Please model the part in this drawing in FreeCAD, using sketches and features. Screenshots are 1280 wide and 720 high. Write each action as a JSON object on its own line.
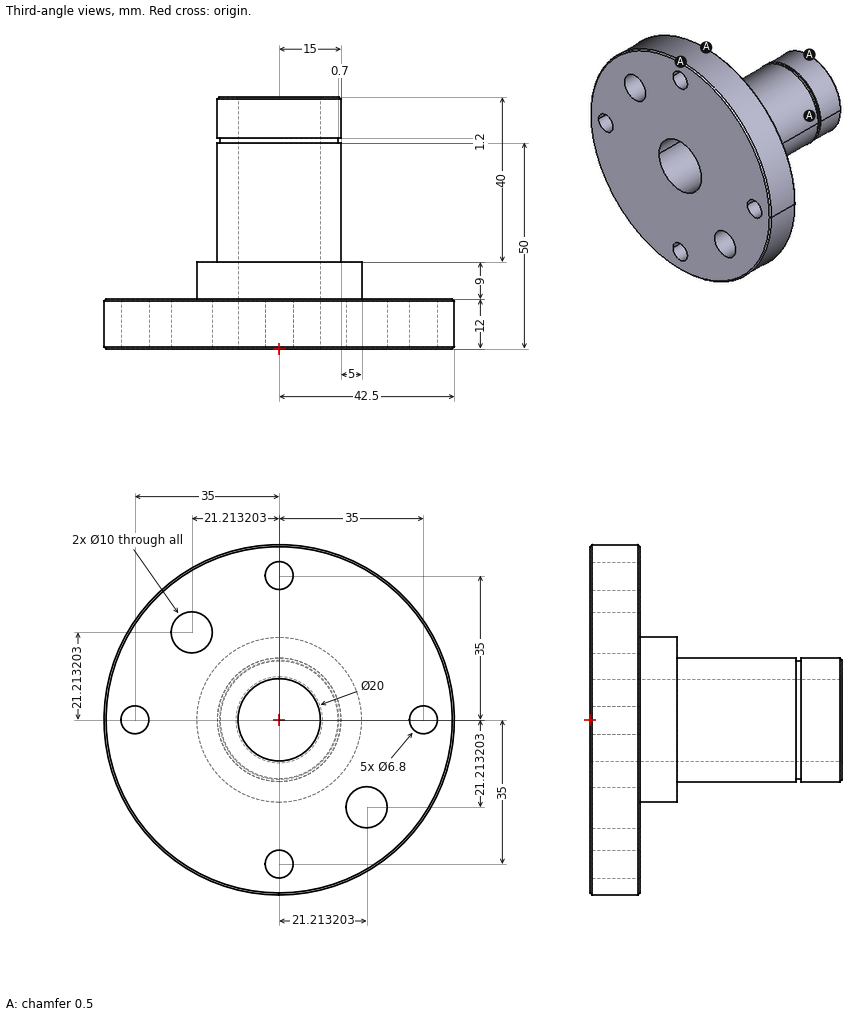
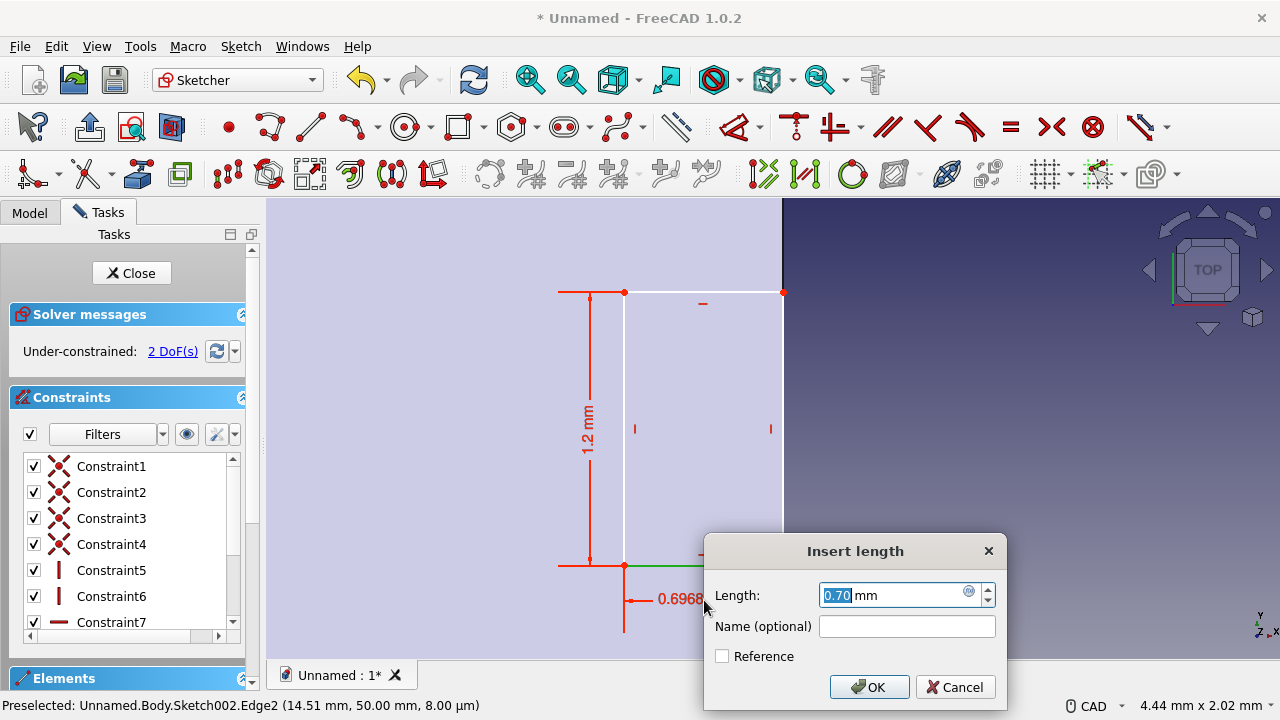
{"action": "type", "text": "0.7"}
{"action": "key", "text": "Return"}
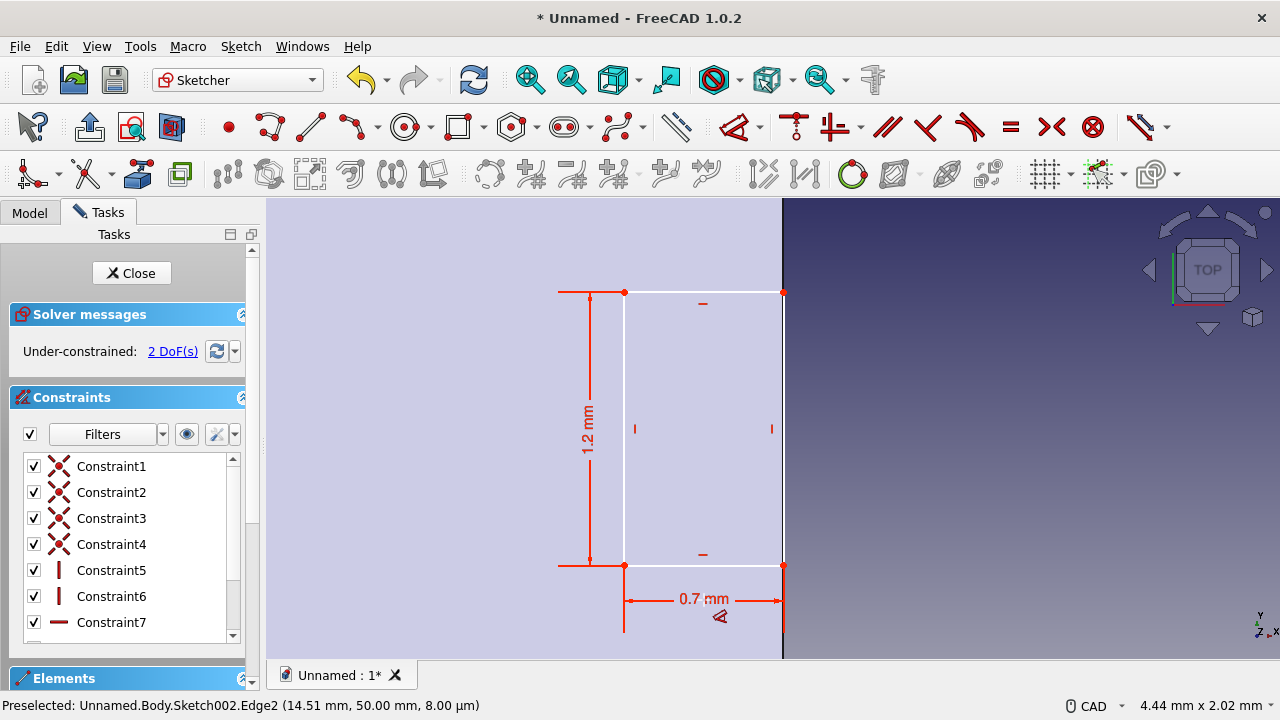
{"action": "left_click", "coordinate": [624, 566]}
{"action": "left_click", "coordinate": [658, 621]}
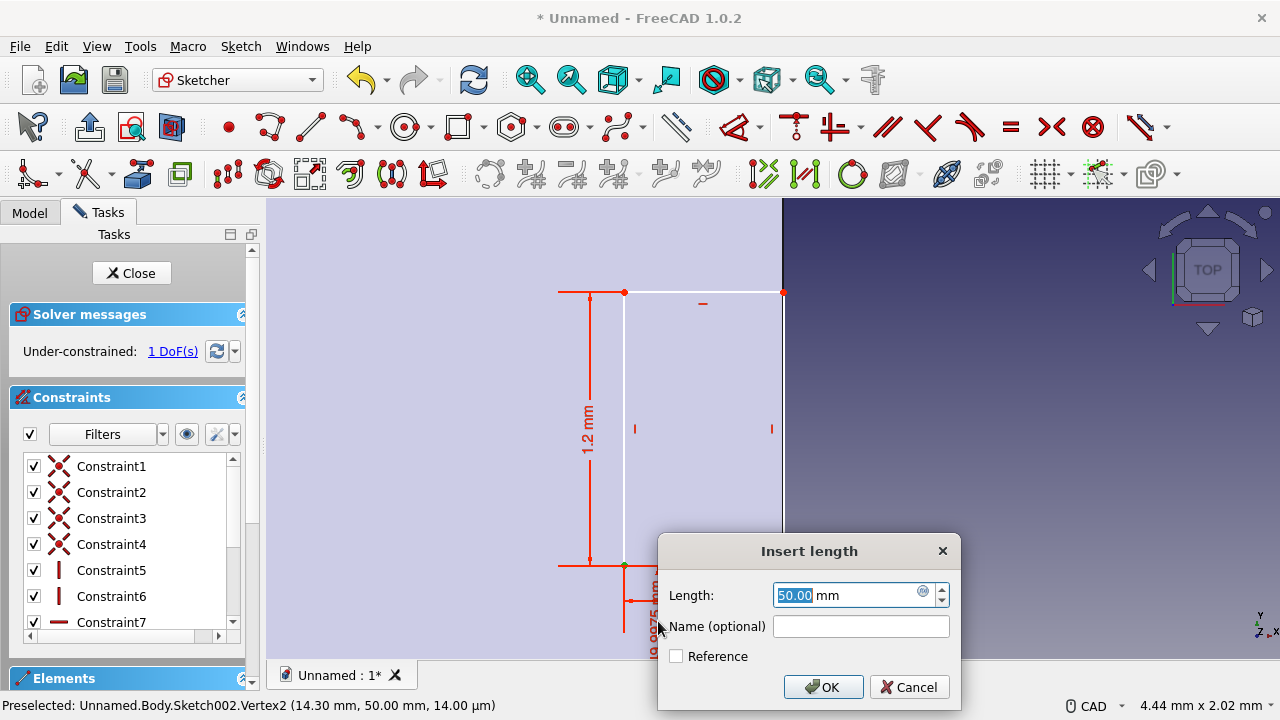
{"action": "type", "text": "50"}
{"action": "key", "text": "Return"}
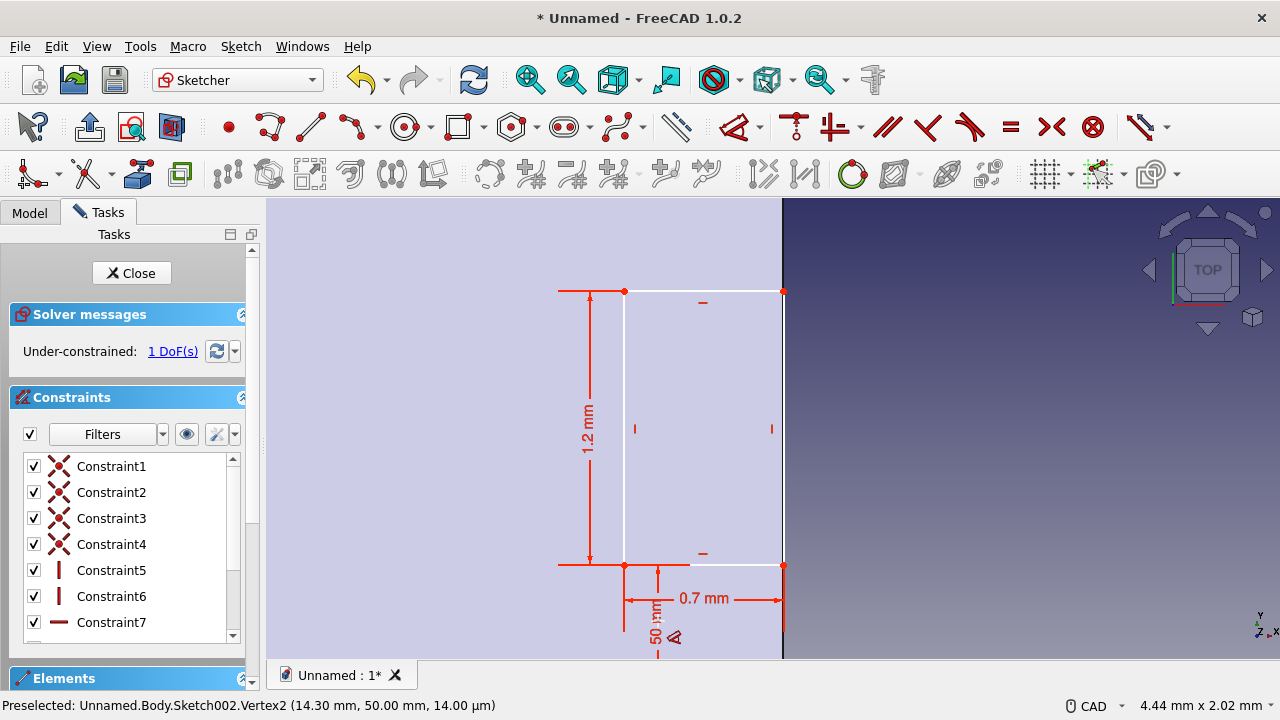
{"action": "left_click", "coordinate": [784, 565]}
{"action": "left_click", "coordinate": [539, 531]}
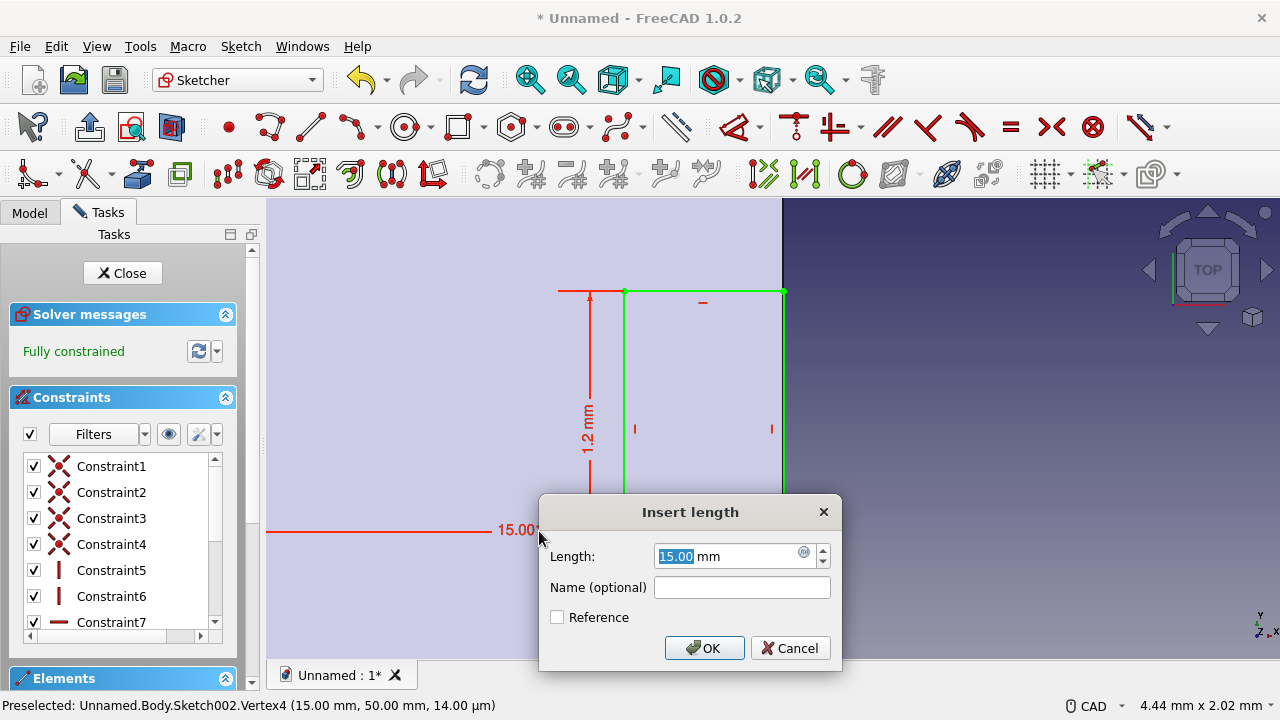
{"action": "type", "text": "15"}
{"action": "key", "text": "Return"}
{"action": "key", "text": "Escape"}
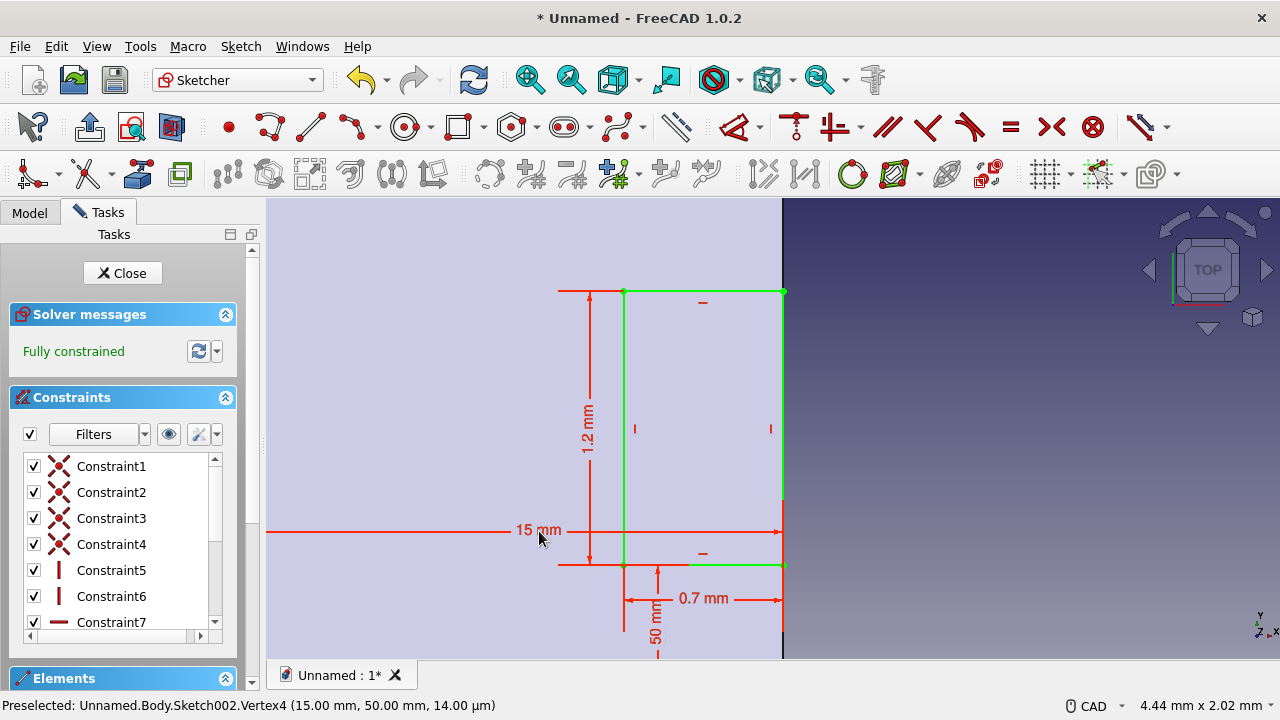
{"action": "left_click", "coordinate": [123, 273]}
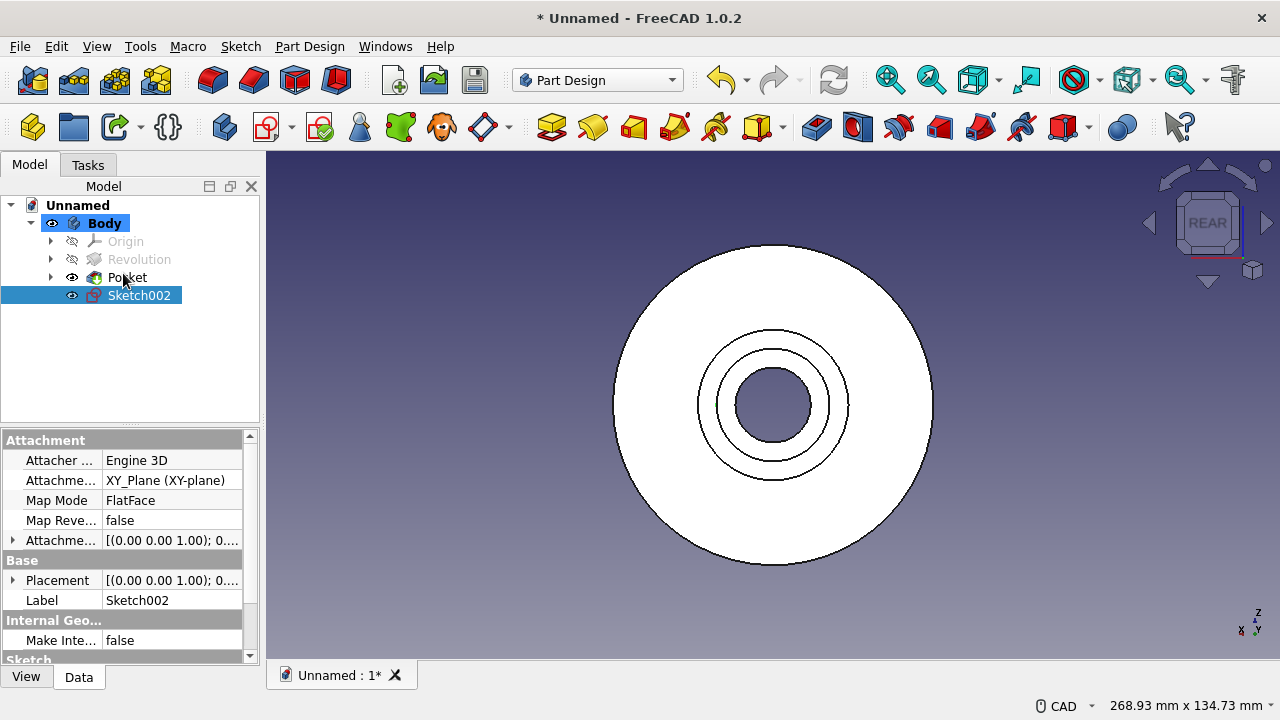
{"action": "left_click", "coordinate": [899, 128]}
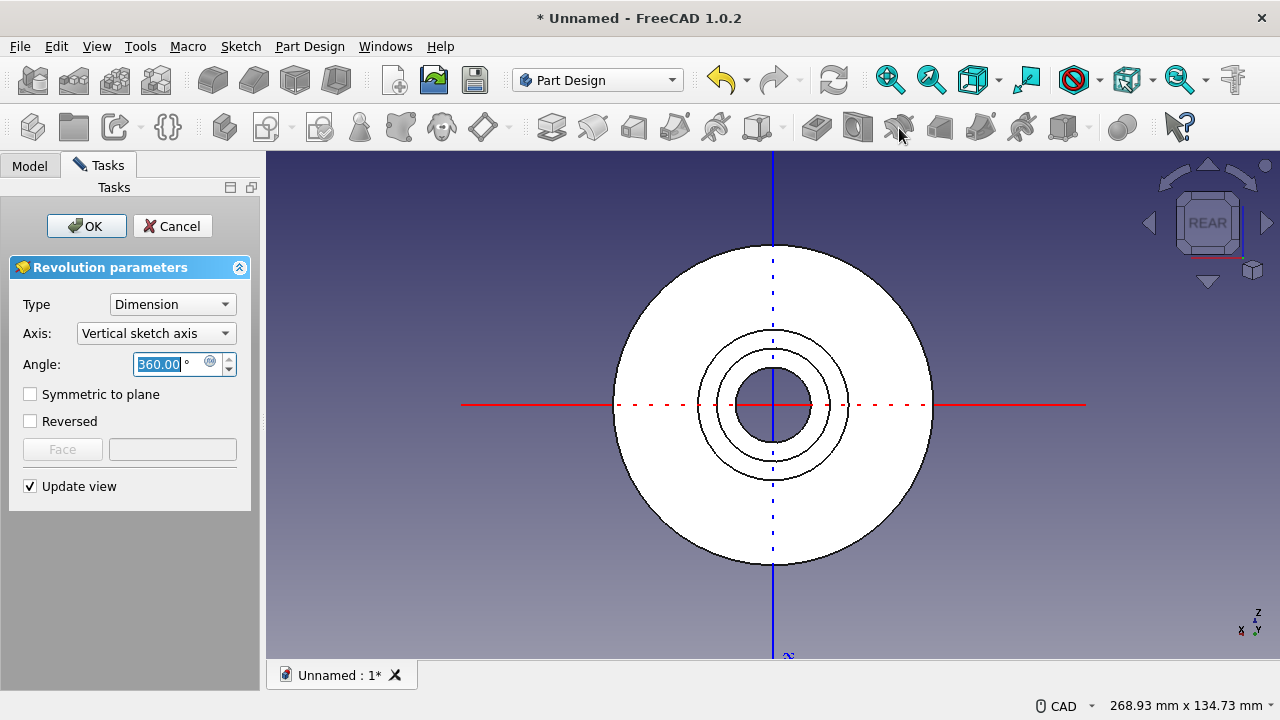
{"action": "left_click", "coordinate": [87, 226]}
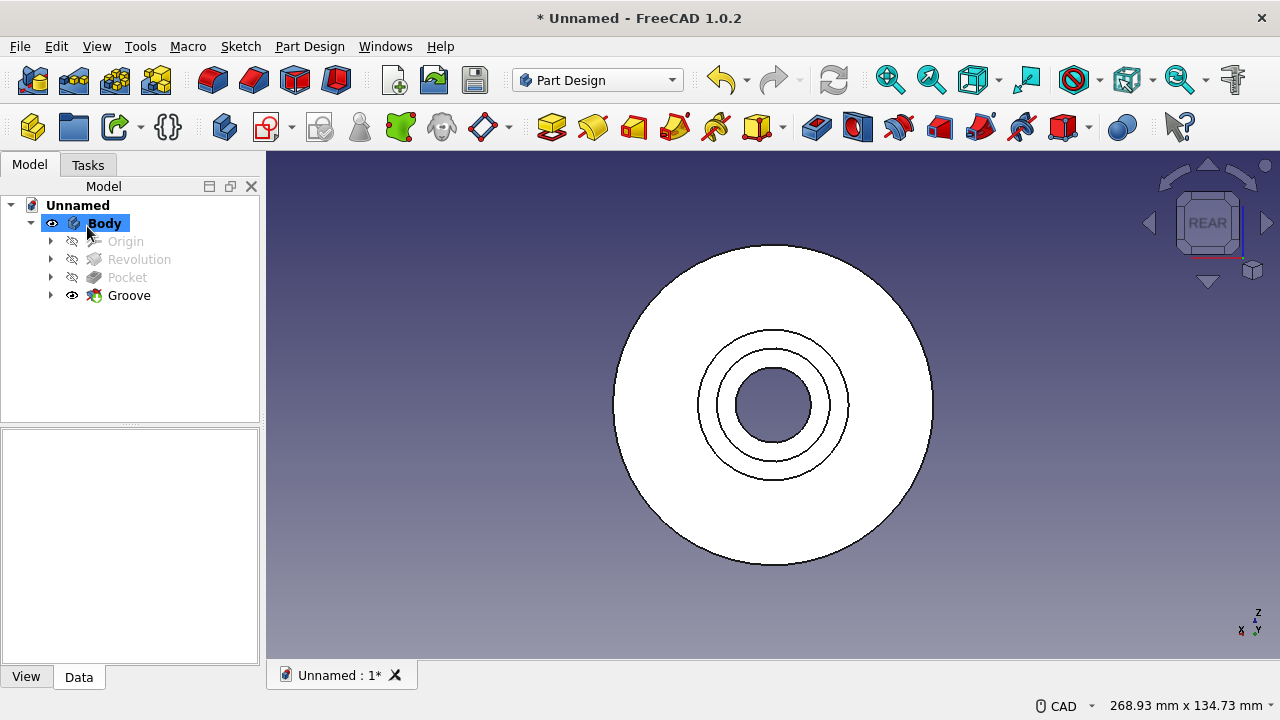
{"action": "left_click", "coordinate": [865, 496]}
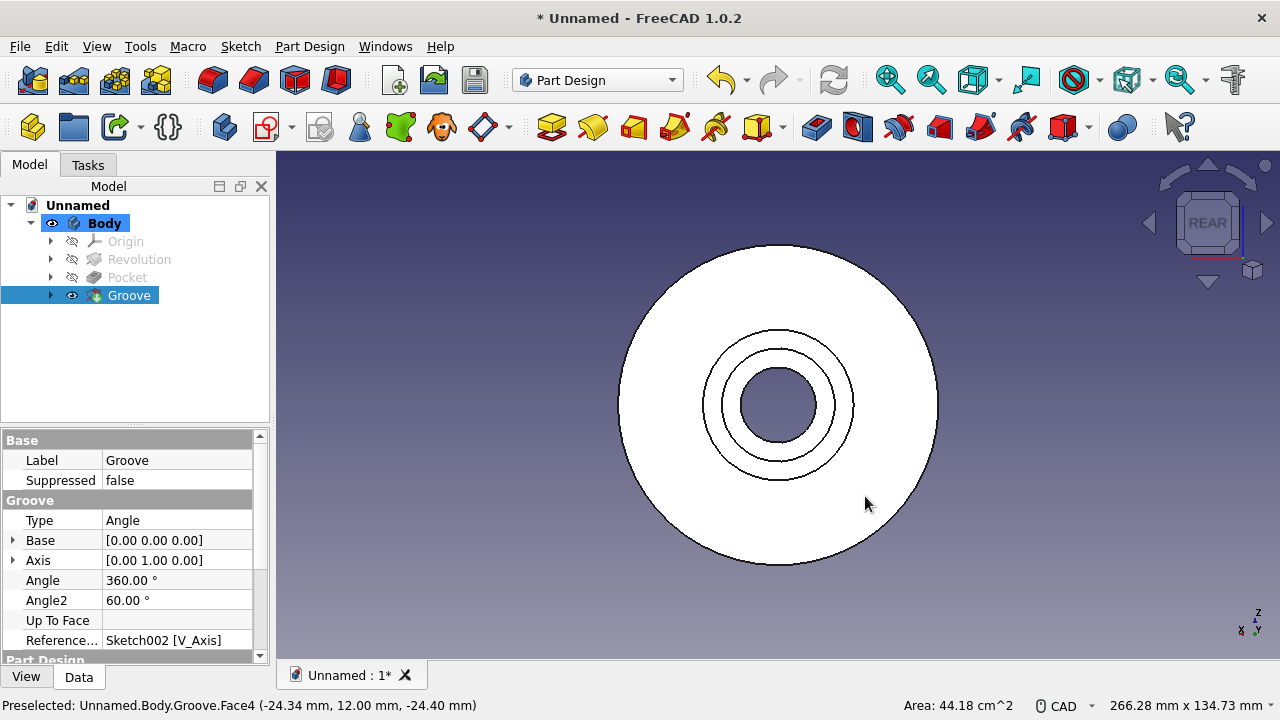
{"action": "left_click", "coordinate": [266, 128]}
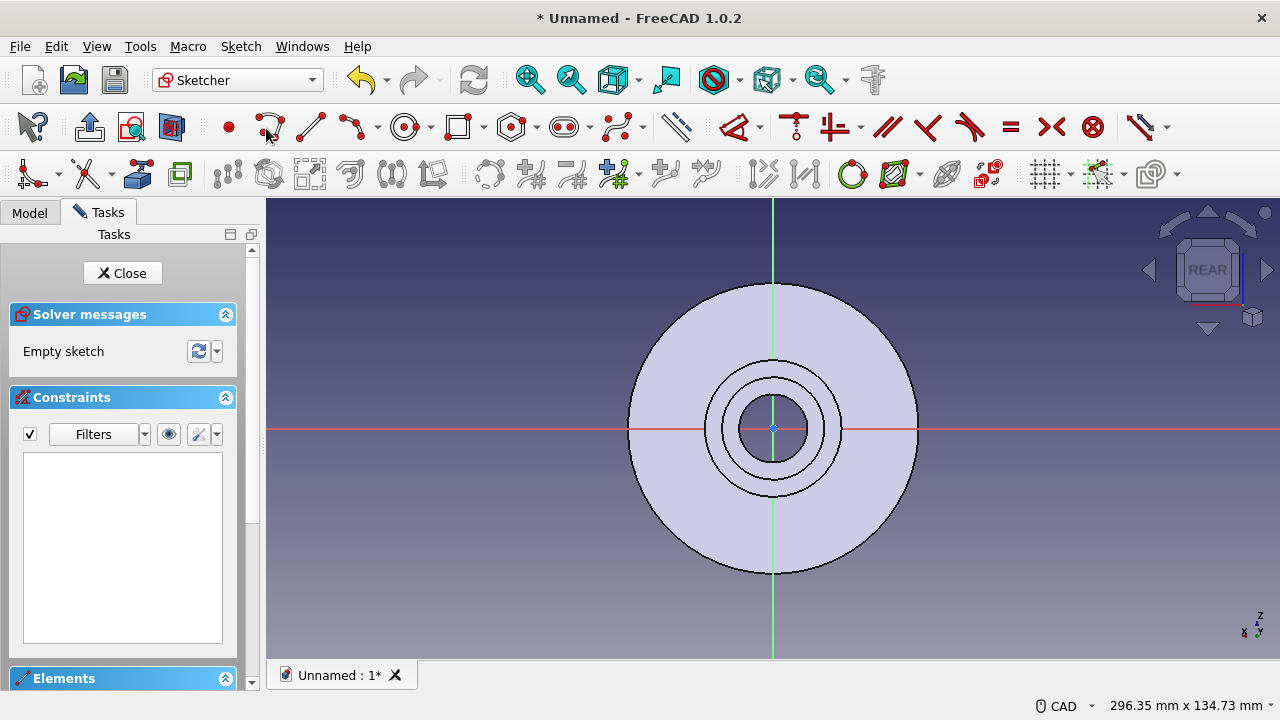
{"action": "key", "text": "q s"}